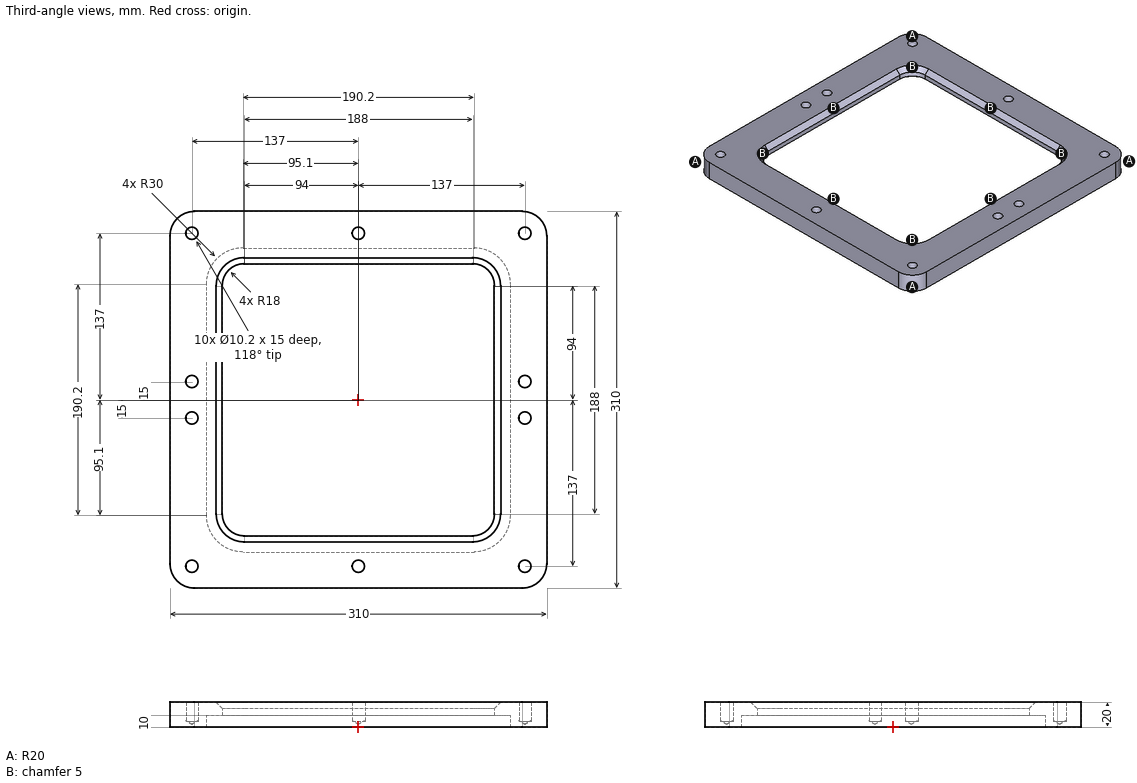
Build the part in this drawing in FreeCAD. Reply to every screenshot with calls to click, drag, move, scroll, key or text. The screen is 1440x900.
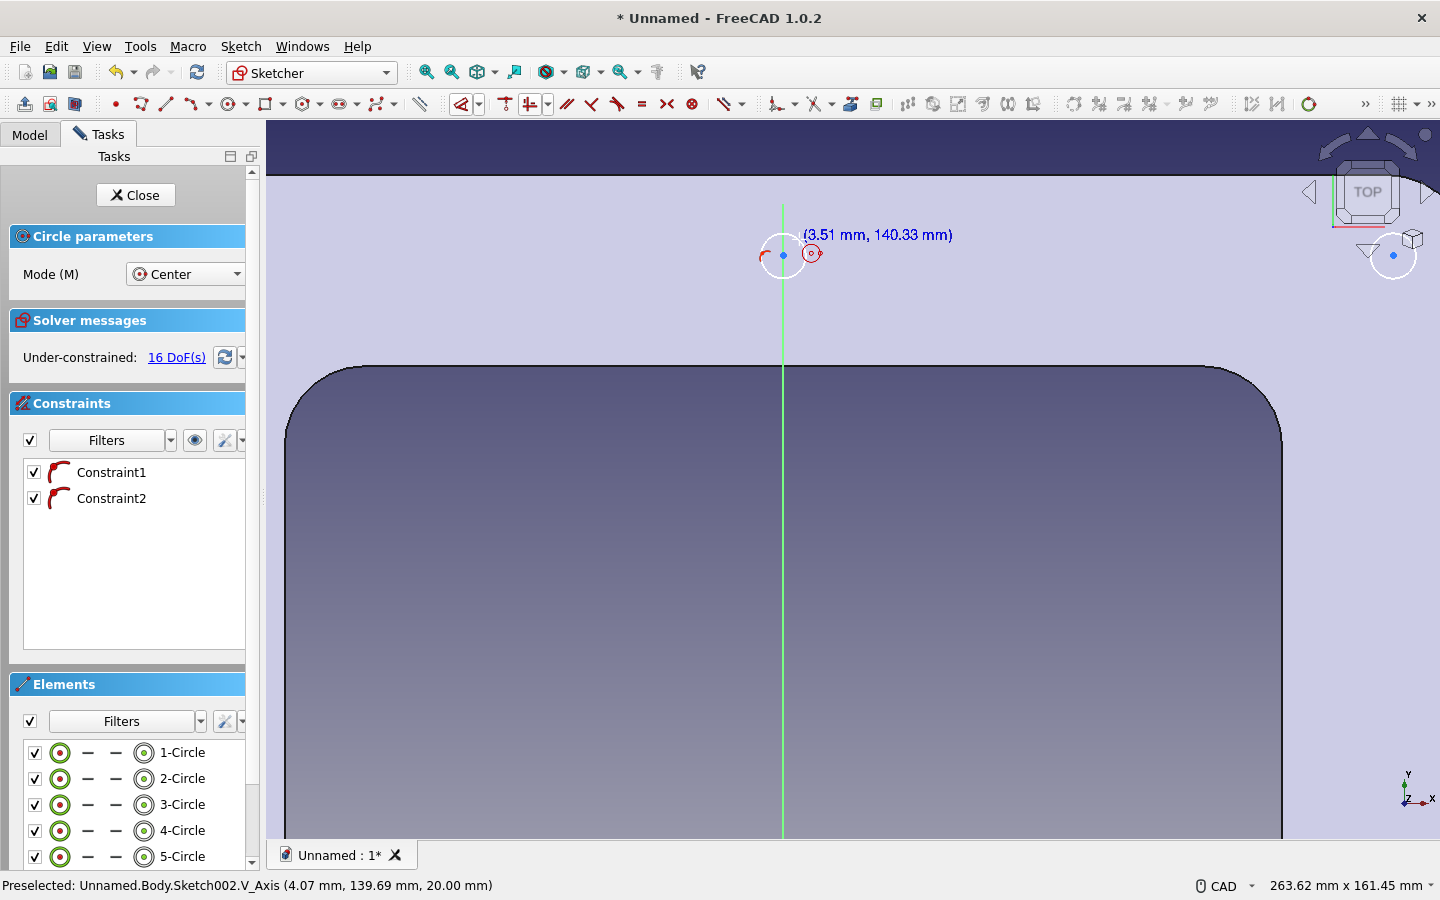
scroll(785, 255, down, 5)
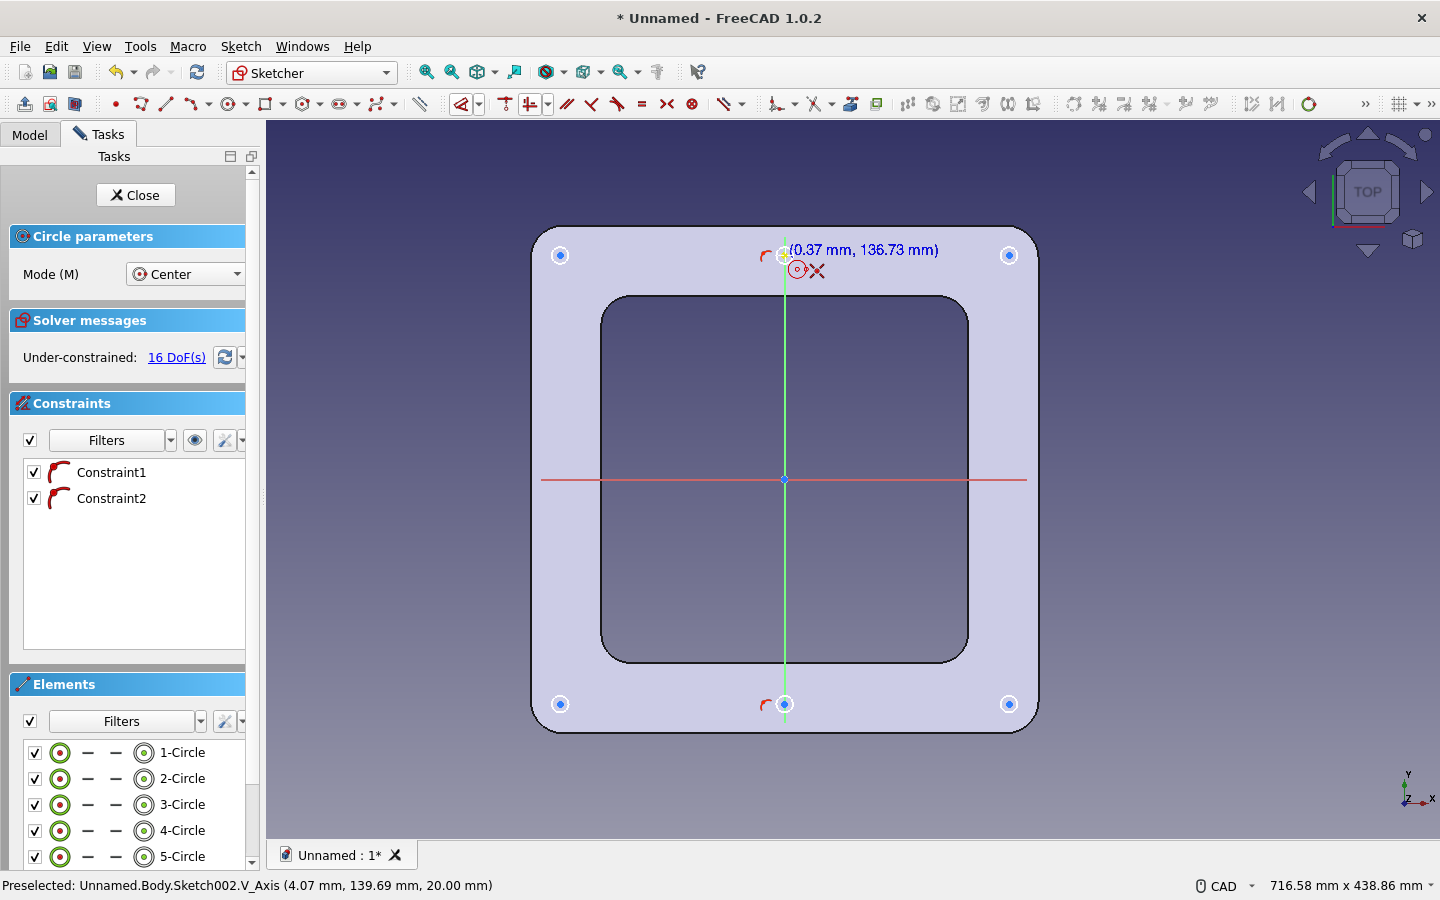
scroll(560, 455, up, 5)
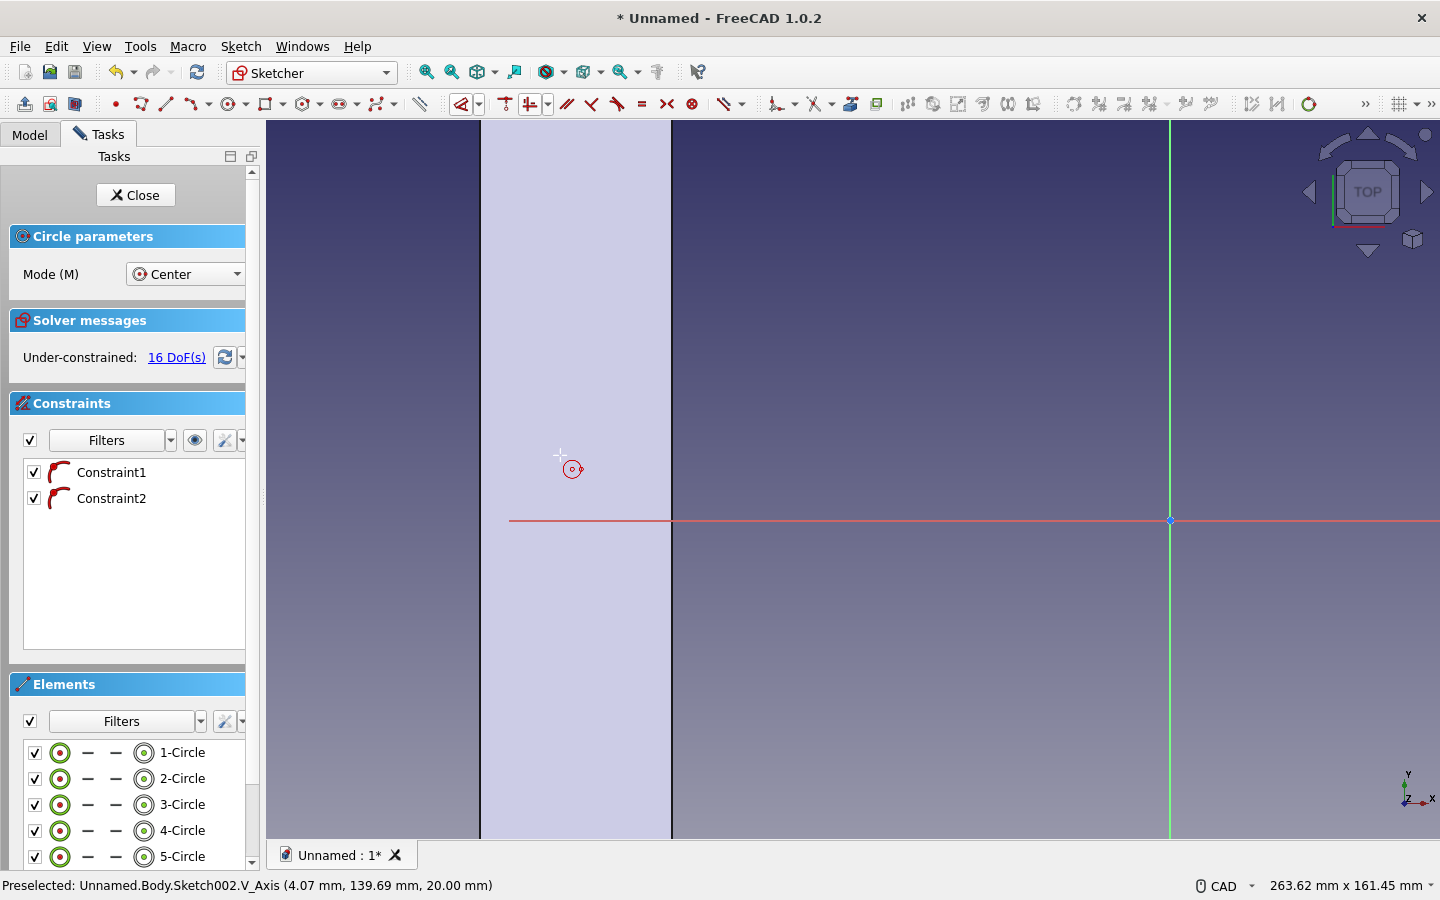
click(560, 454)
click(576, 438)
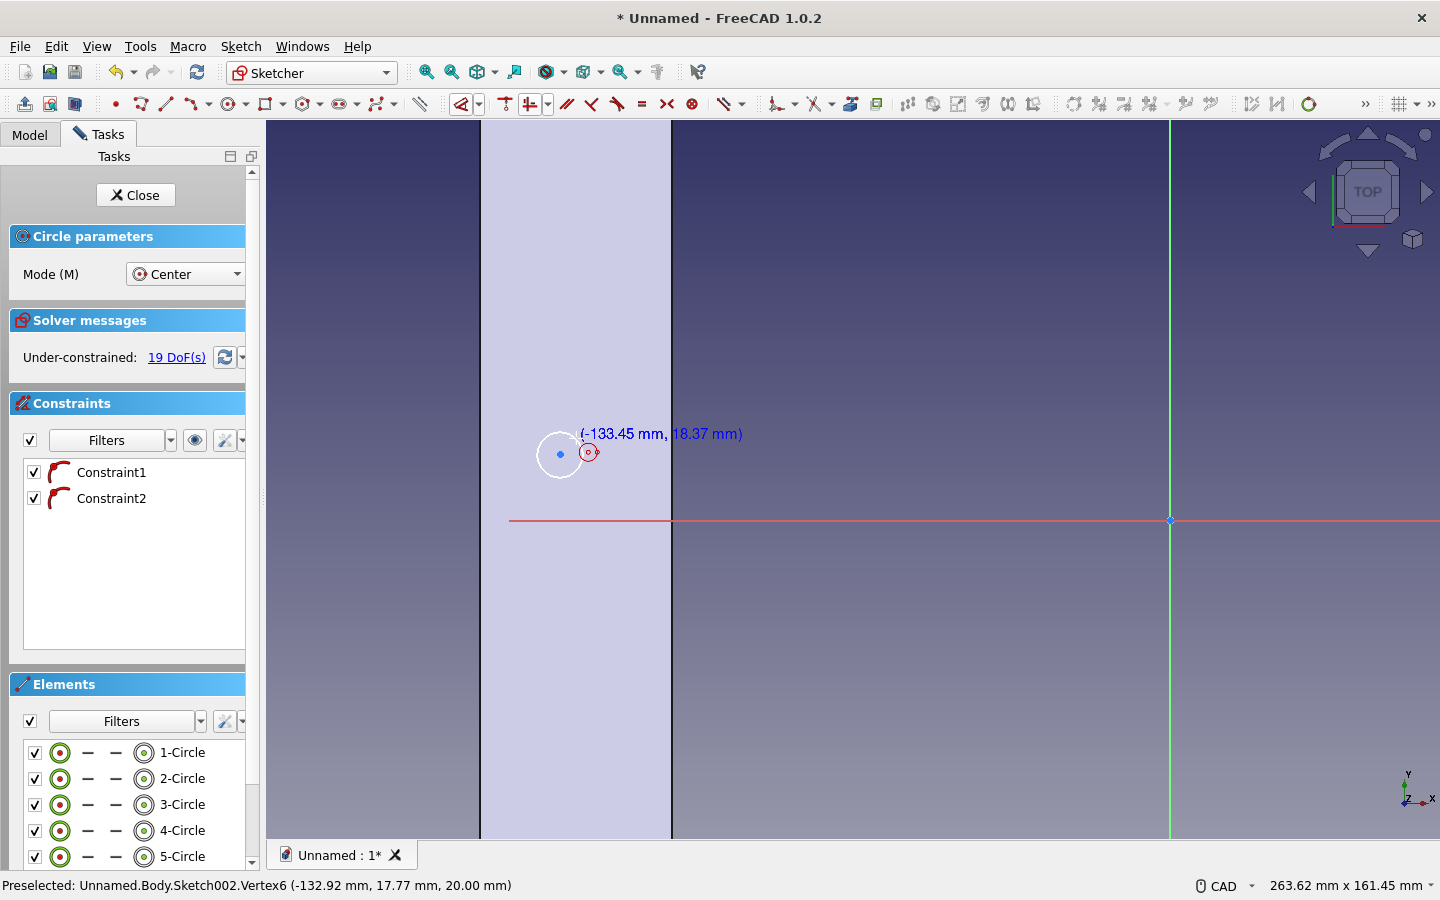
click(560, 588)
click(576, 572)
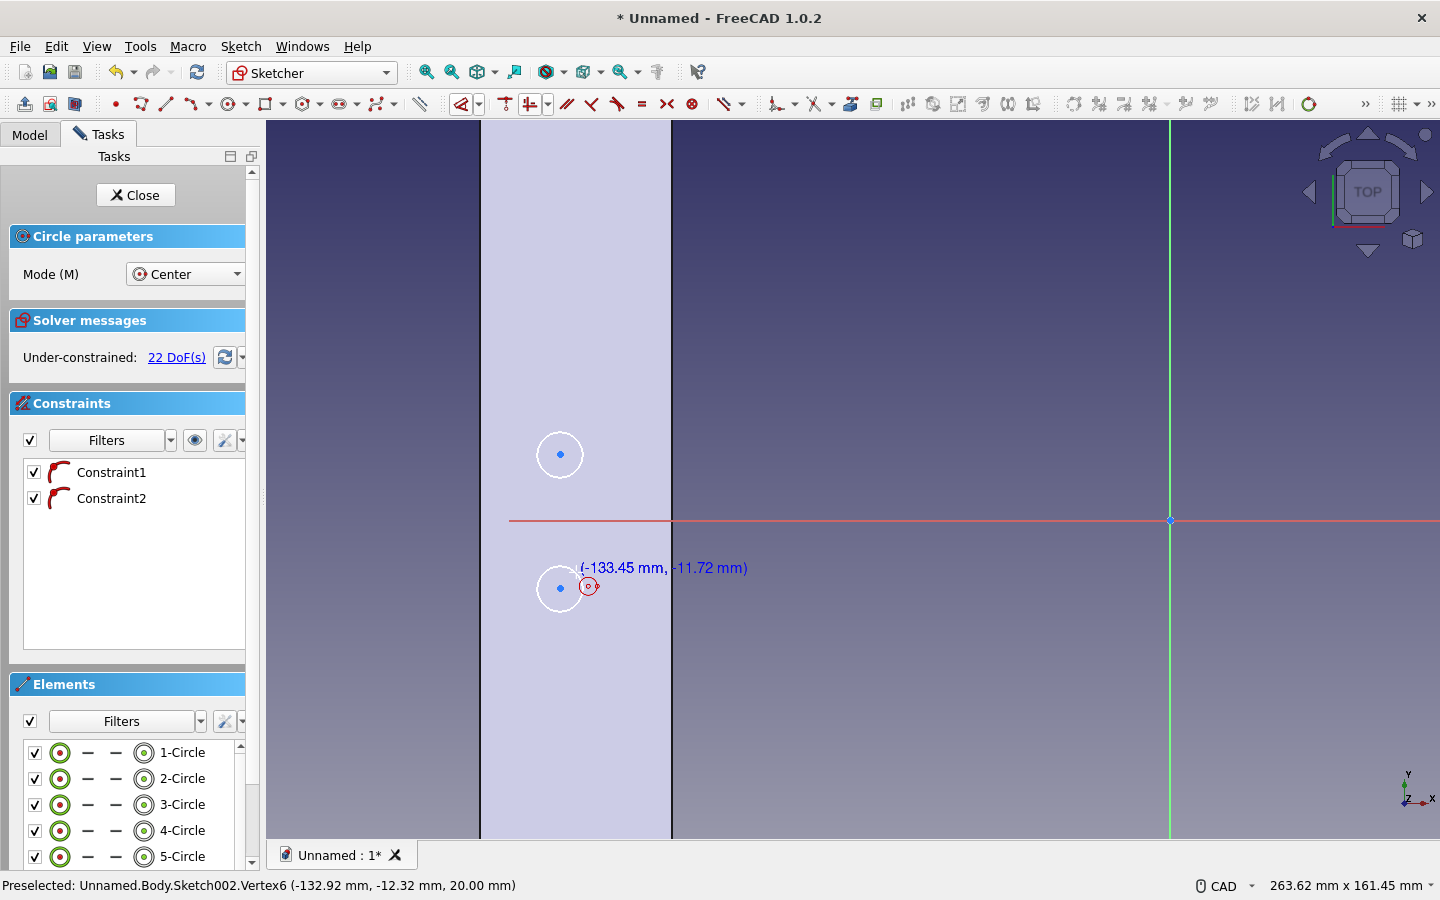
scroll(560, 455, down, 5)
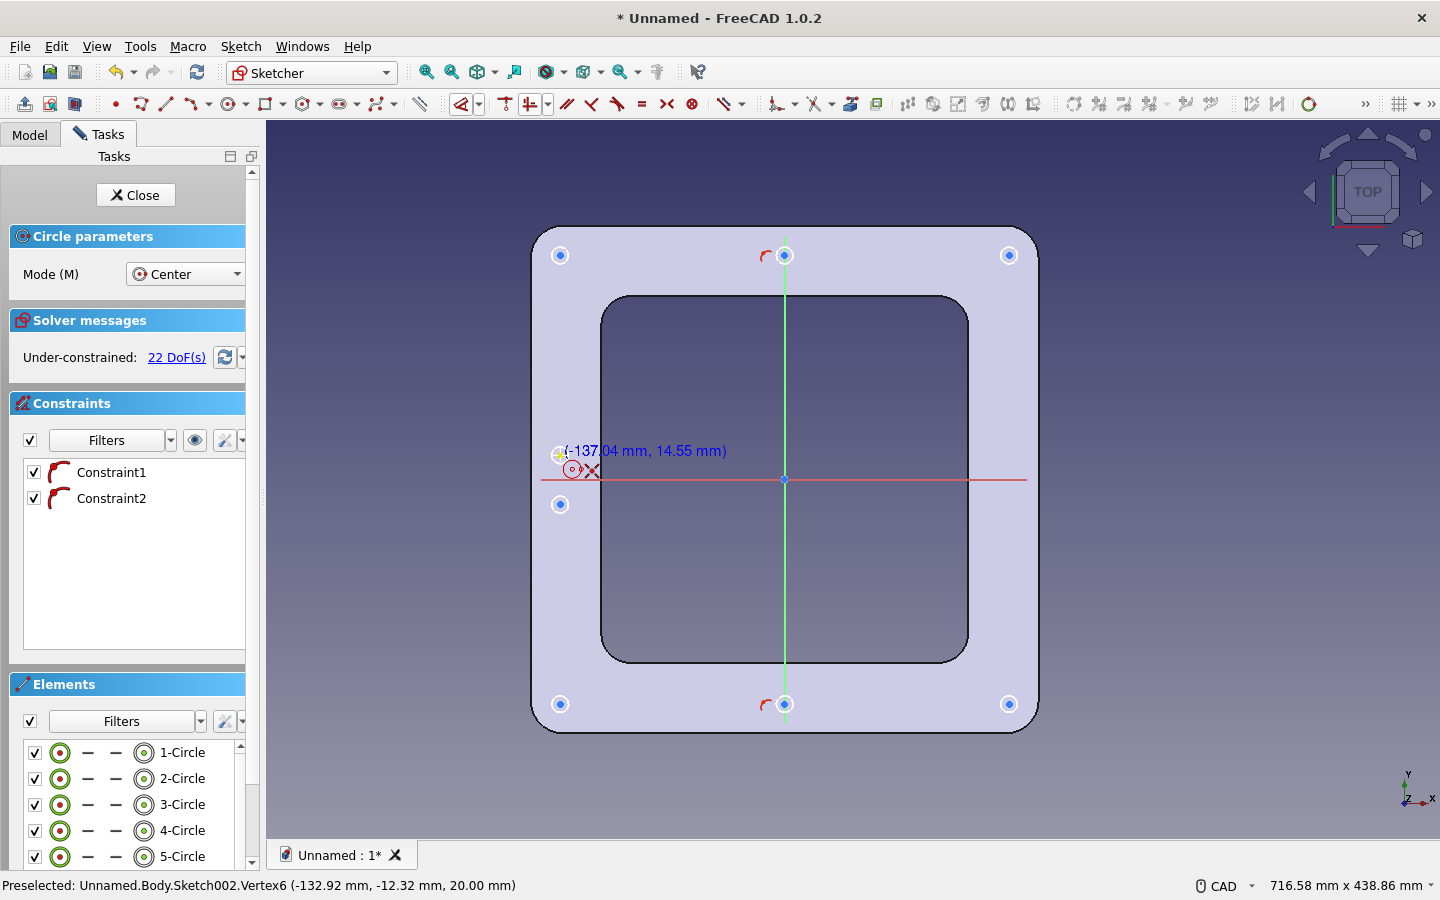
scroll(1009, 455, up, 5)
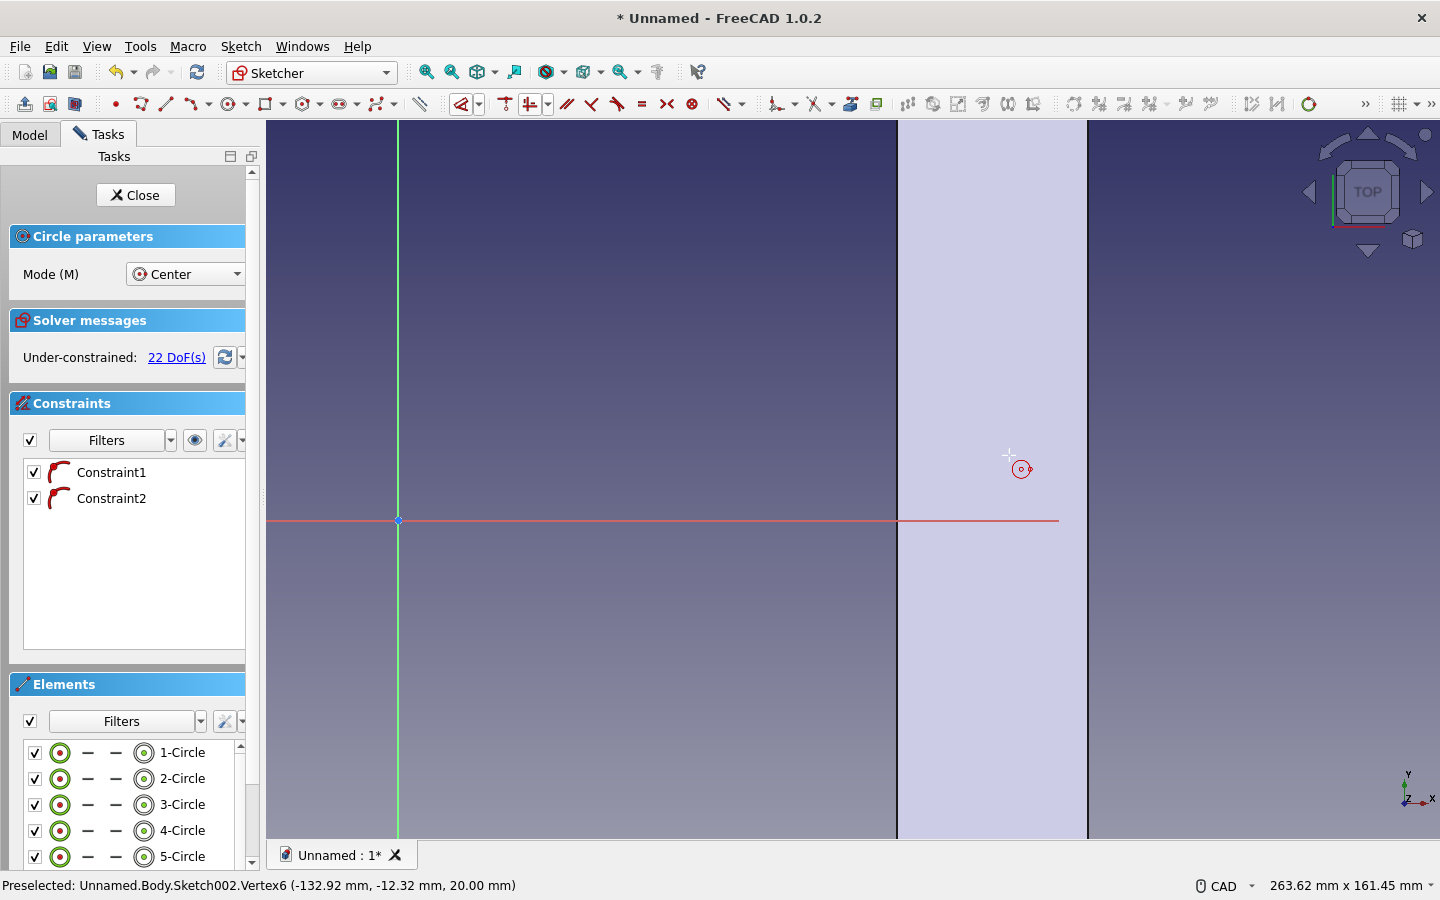
click(1008, 454)
click(1024, 438)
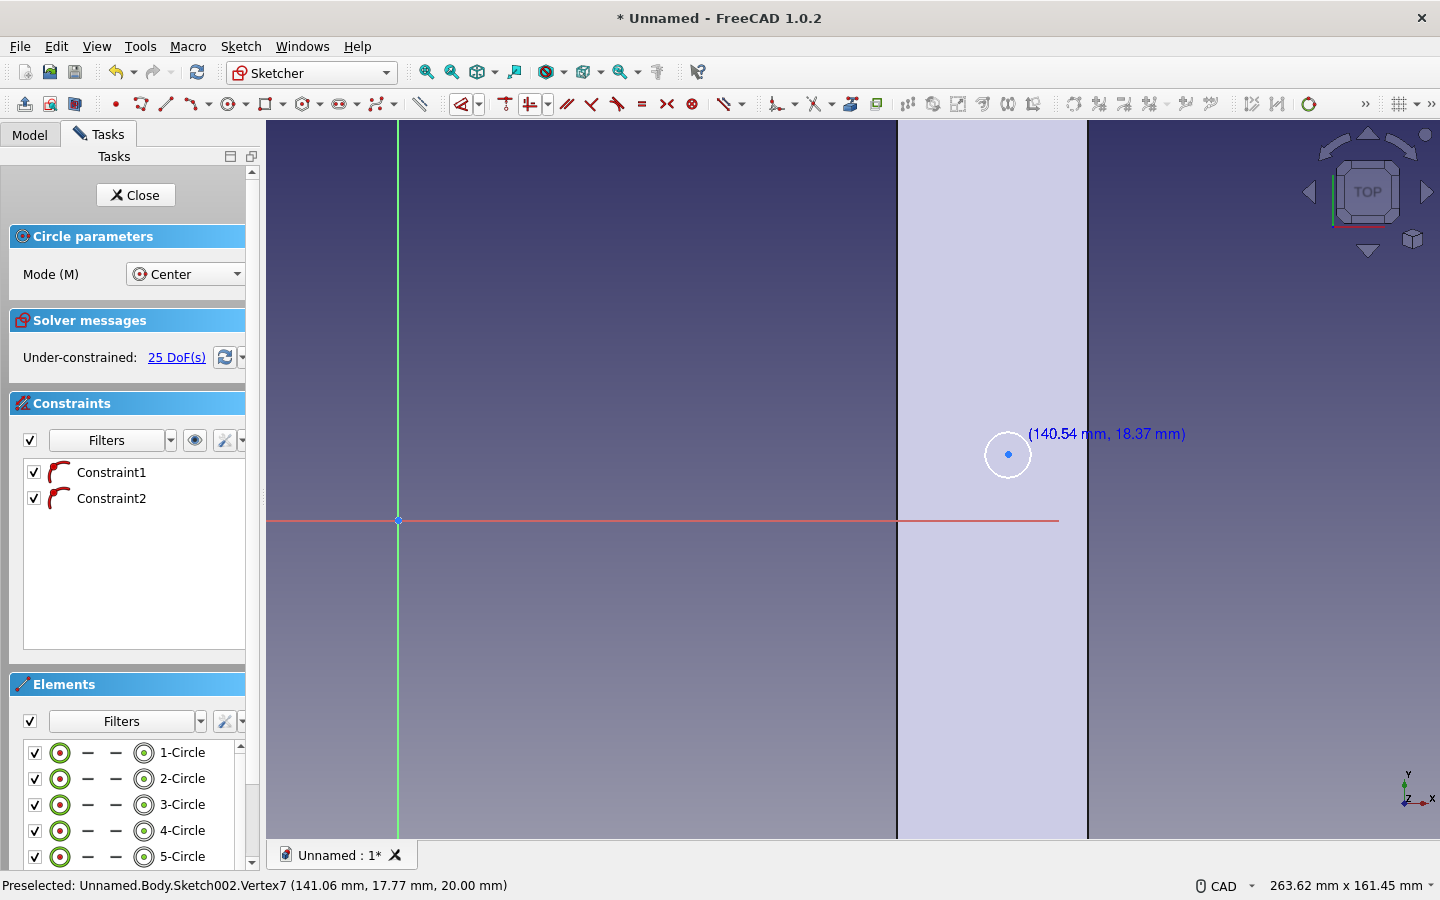
click(1008, 588)
click(1024, 572)
key(Escape)